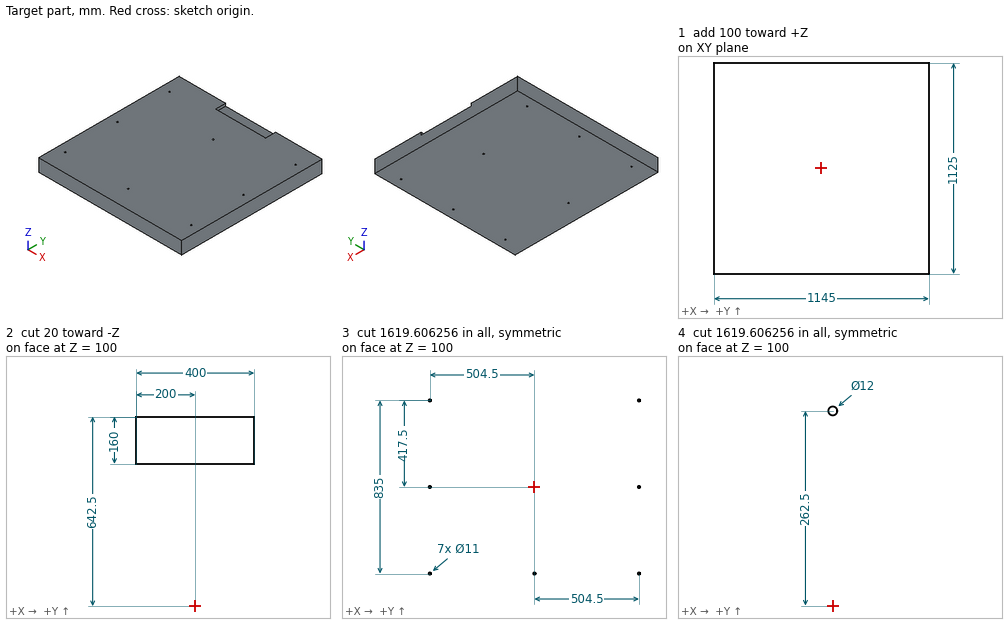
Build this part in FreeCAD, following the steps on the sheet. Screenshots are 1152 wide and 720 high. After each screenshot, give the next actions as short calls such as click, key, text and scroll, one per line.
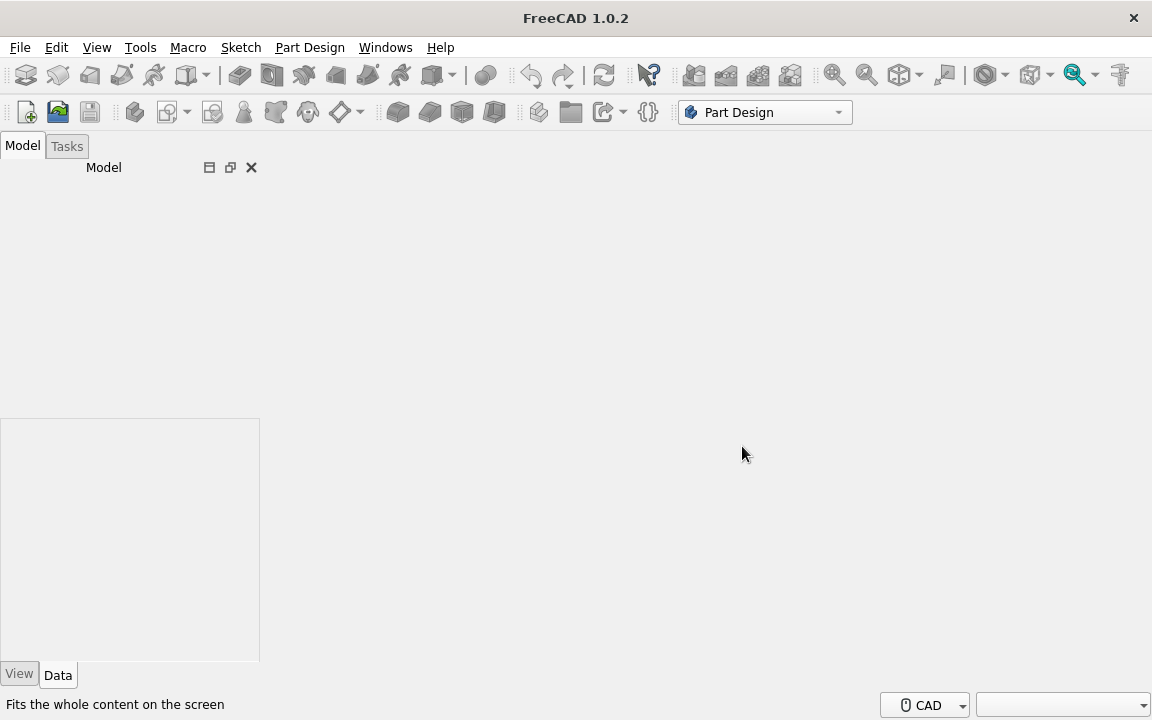
click(26, 112)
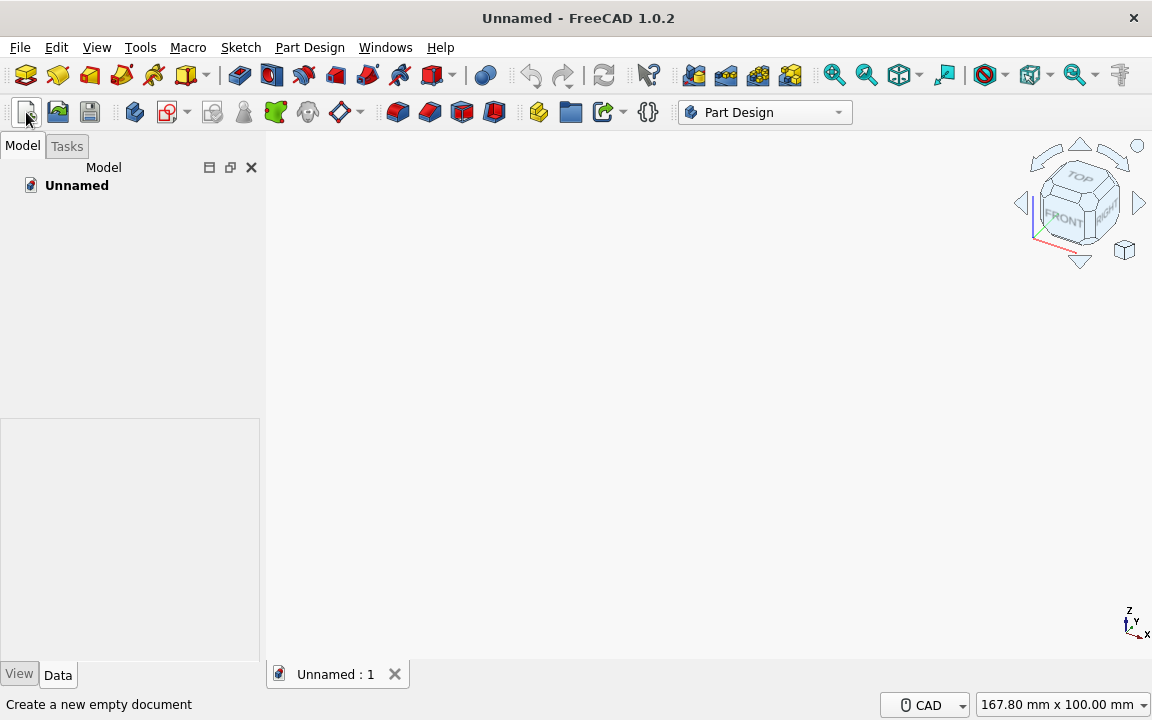
click(168, 112)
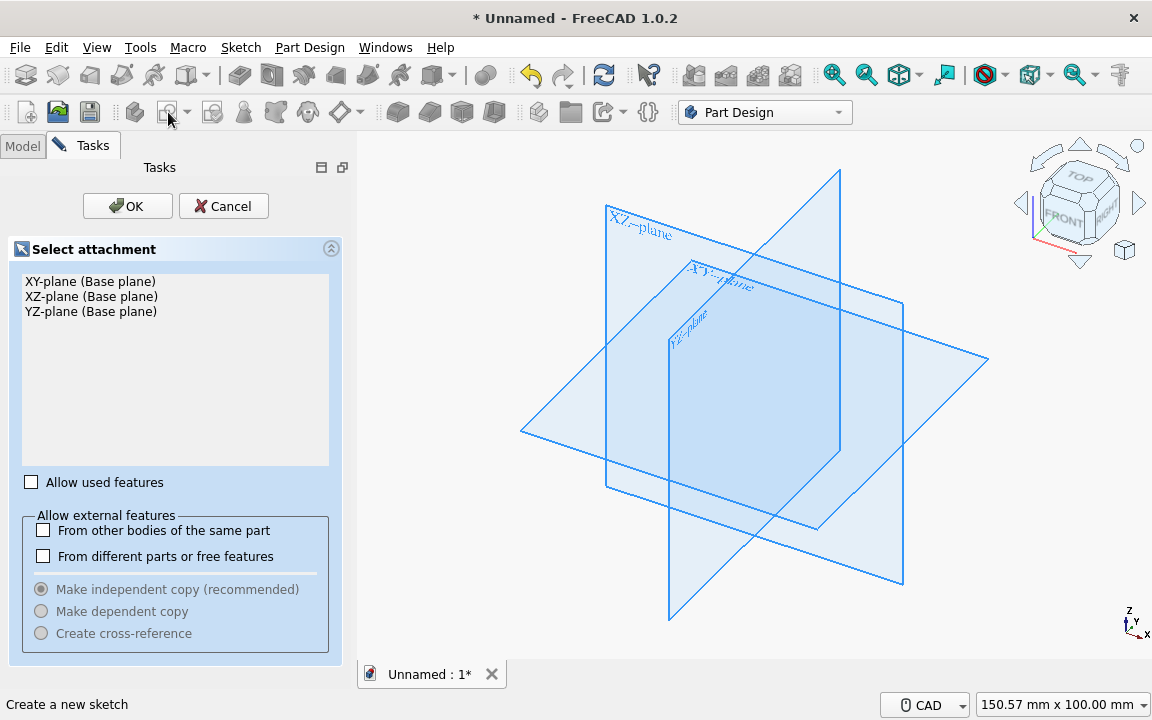
click(82, 282)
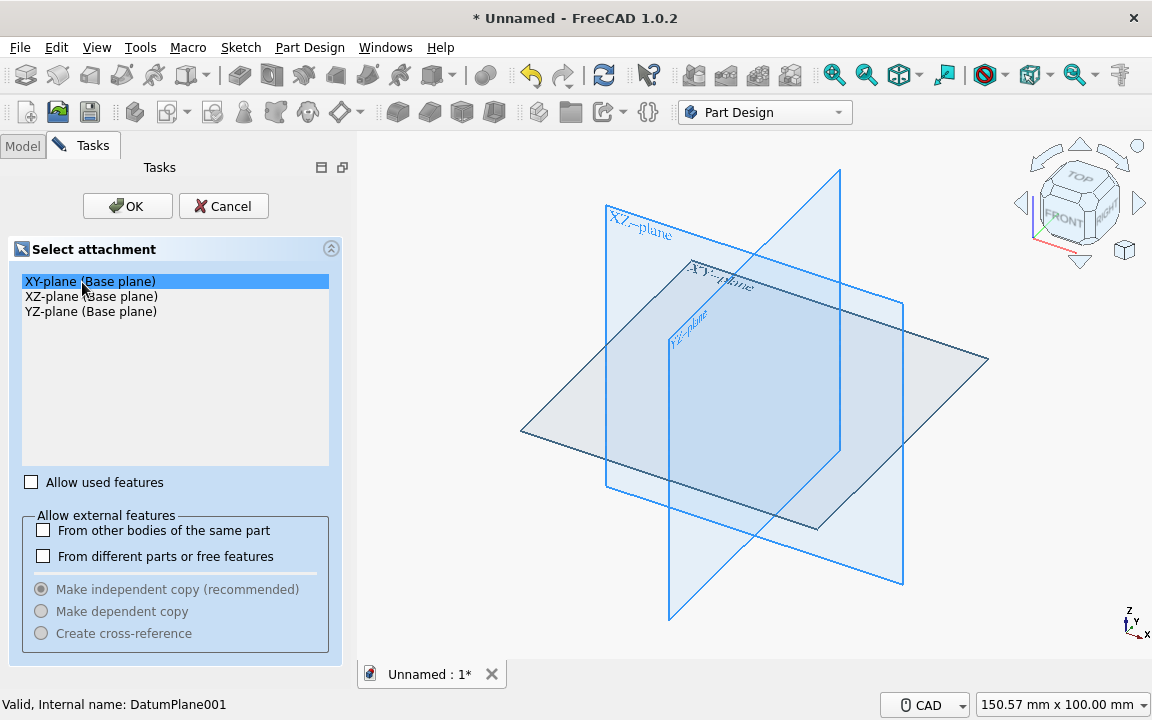
click(128, 206)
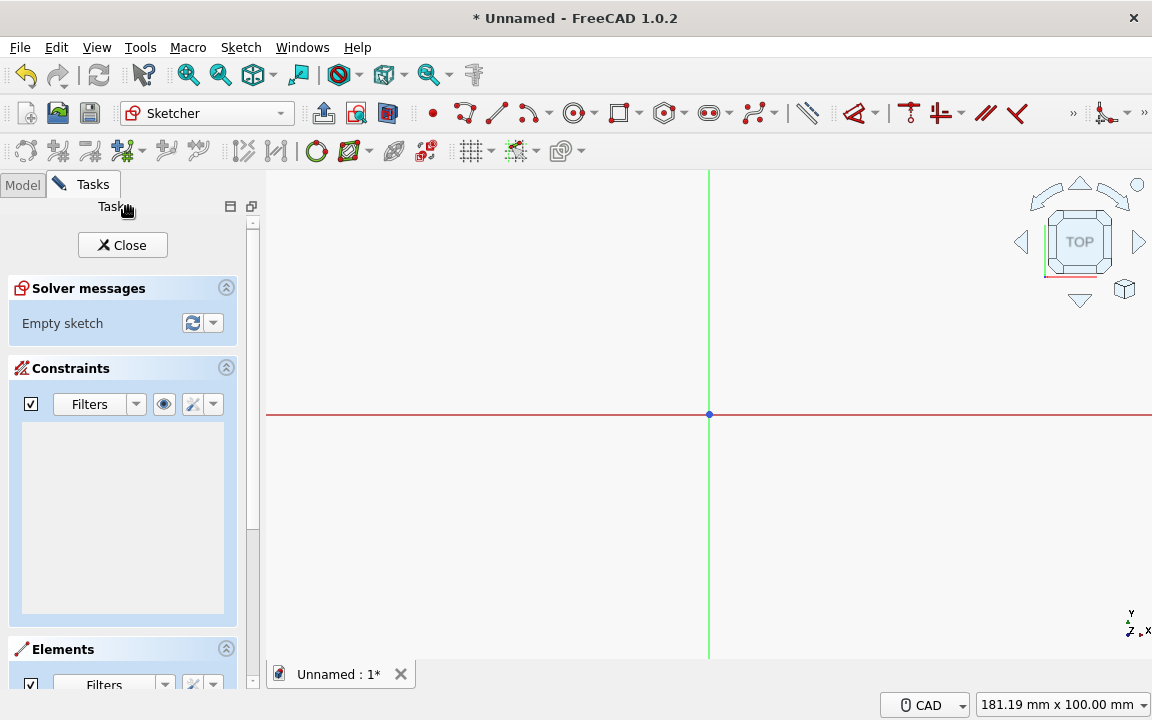
scroll(636, 414, down, 14)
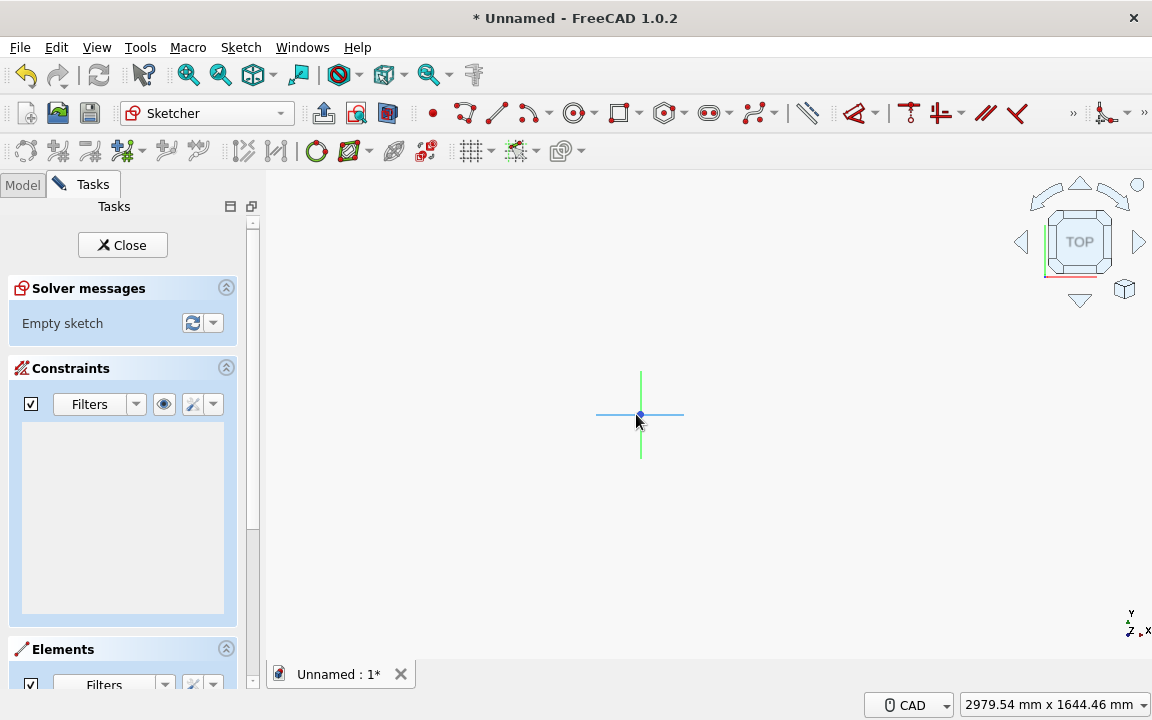
click(642, 114)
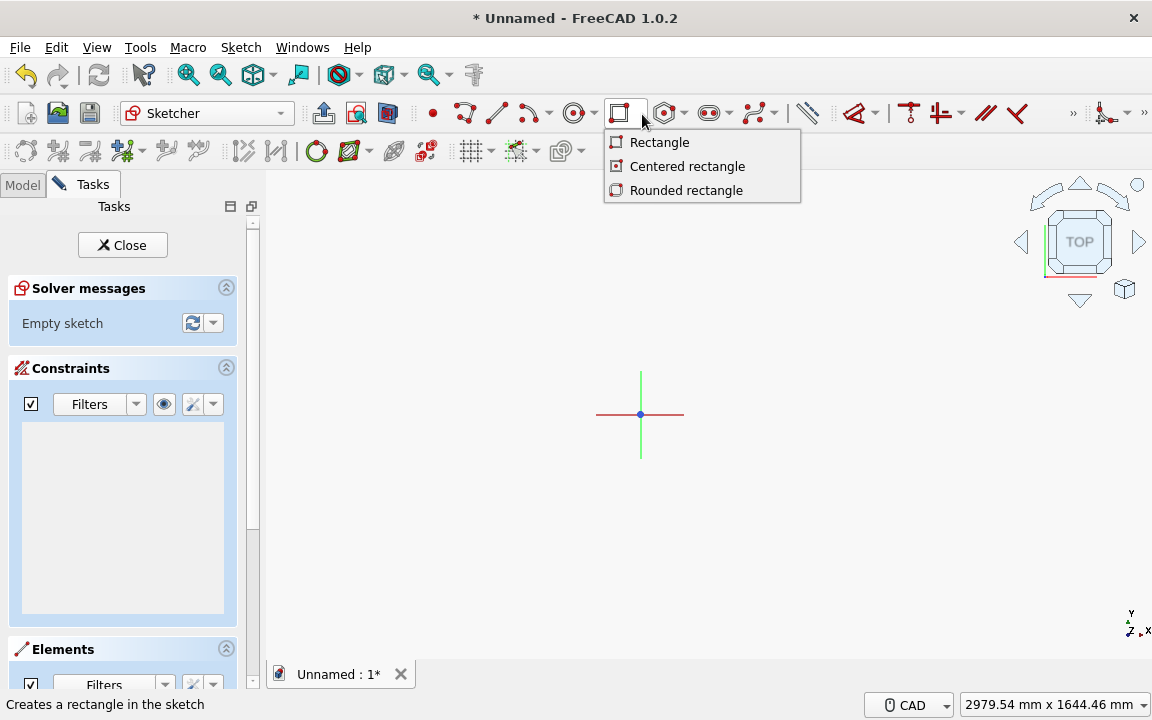
click(702, 166)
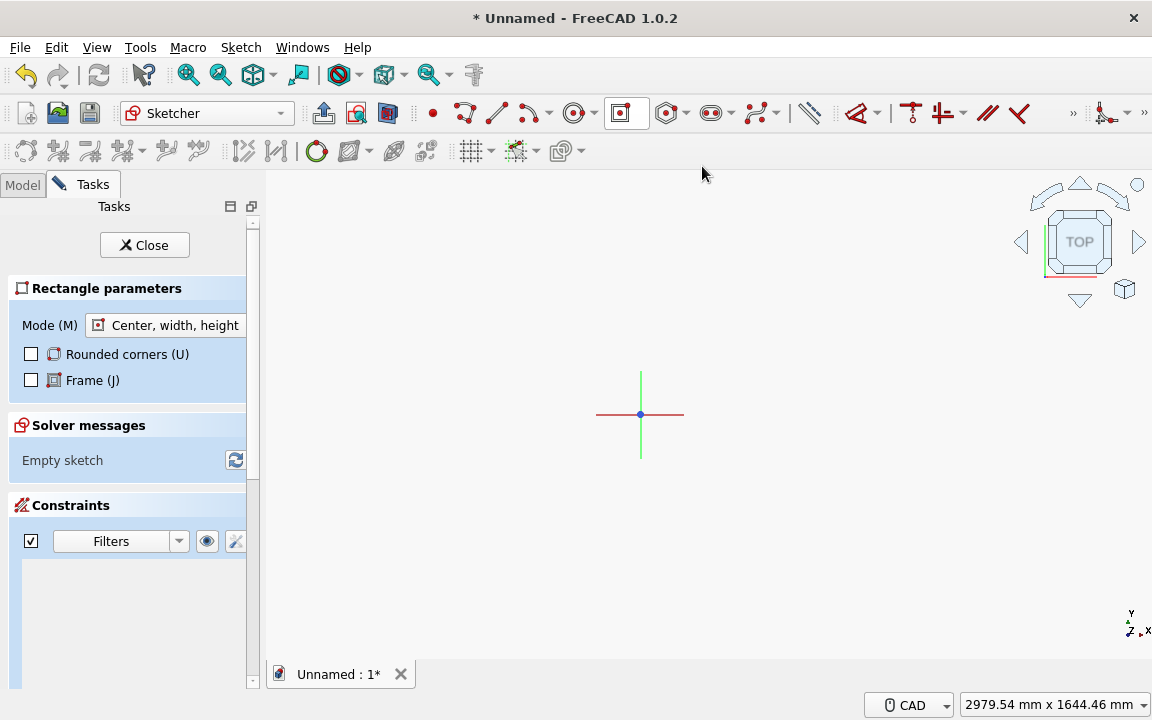
click(641, 414)
click(811, 247)
key(Escape)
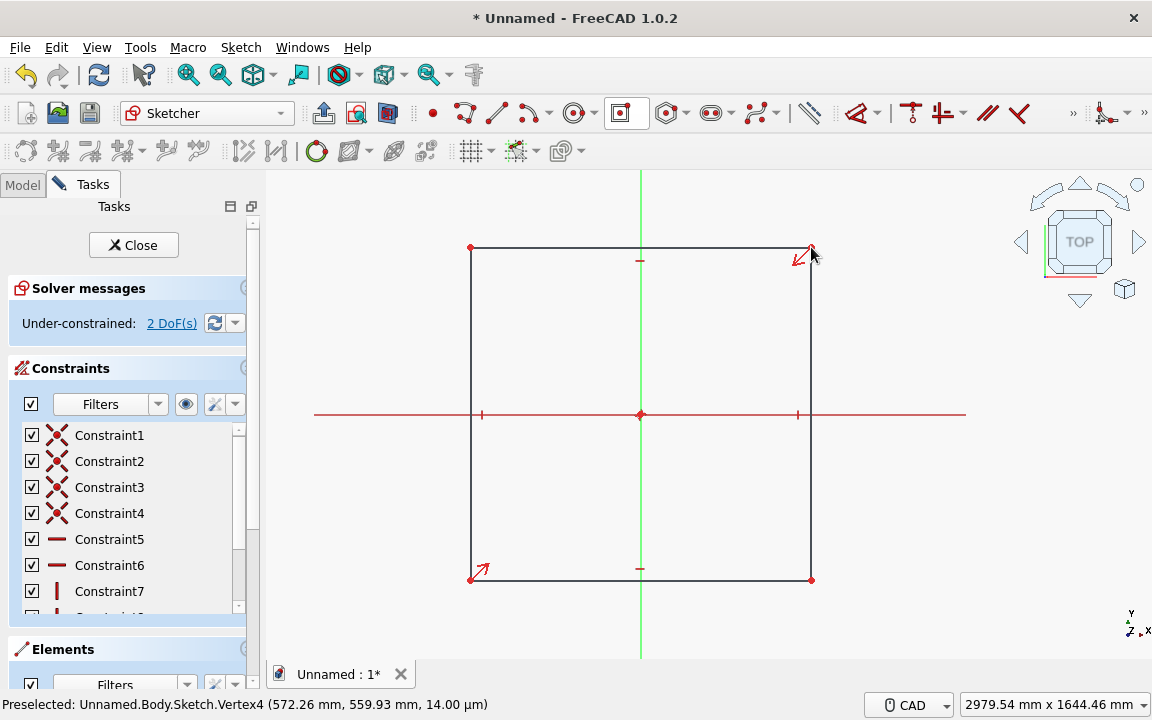
key(d)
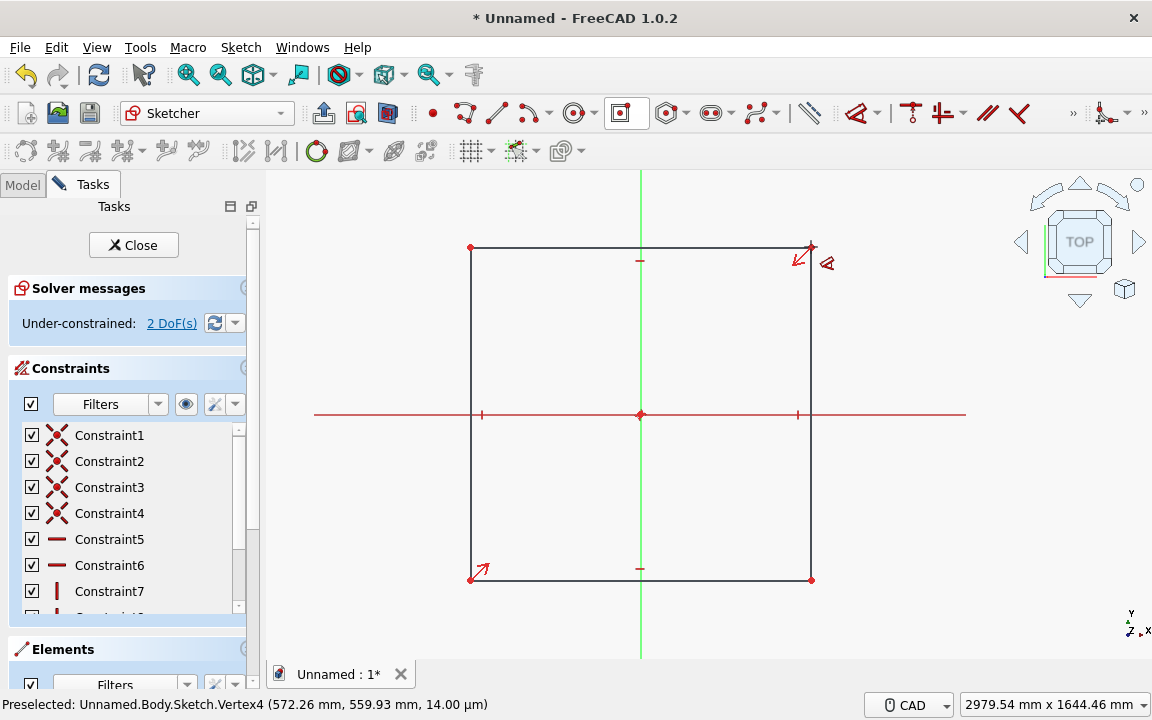
click(573, 581)
click(563, 615)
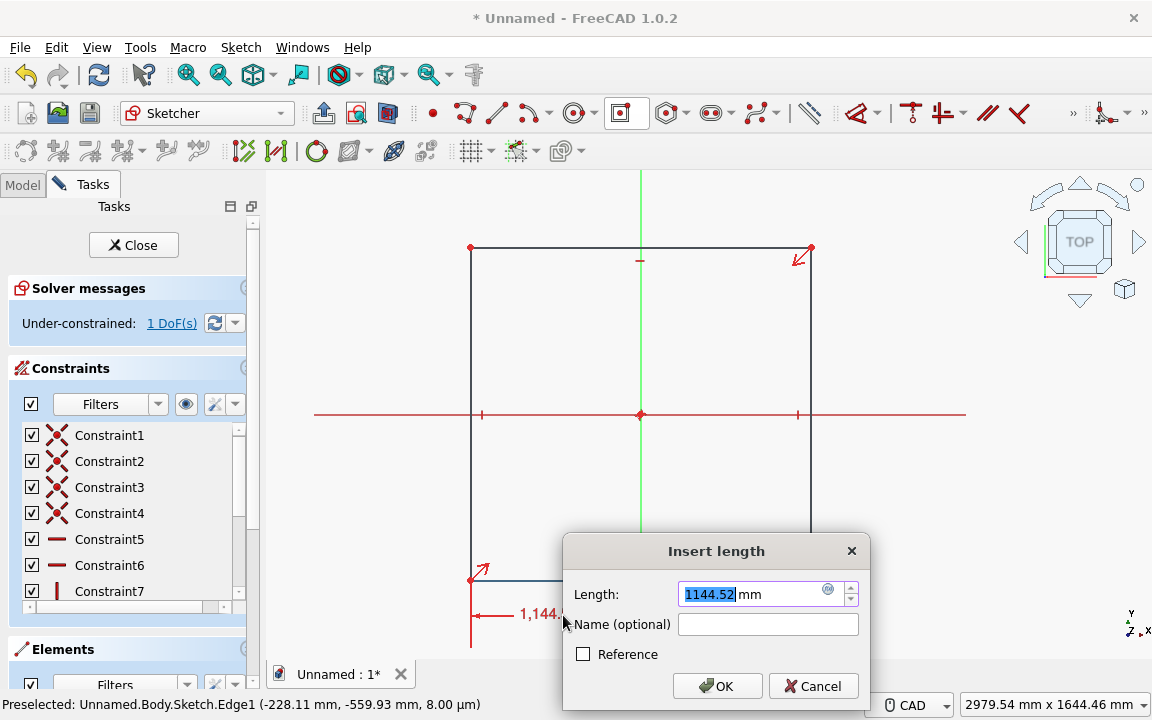
text(1145)
key(Return)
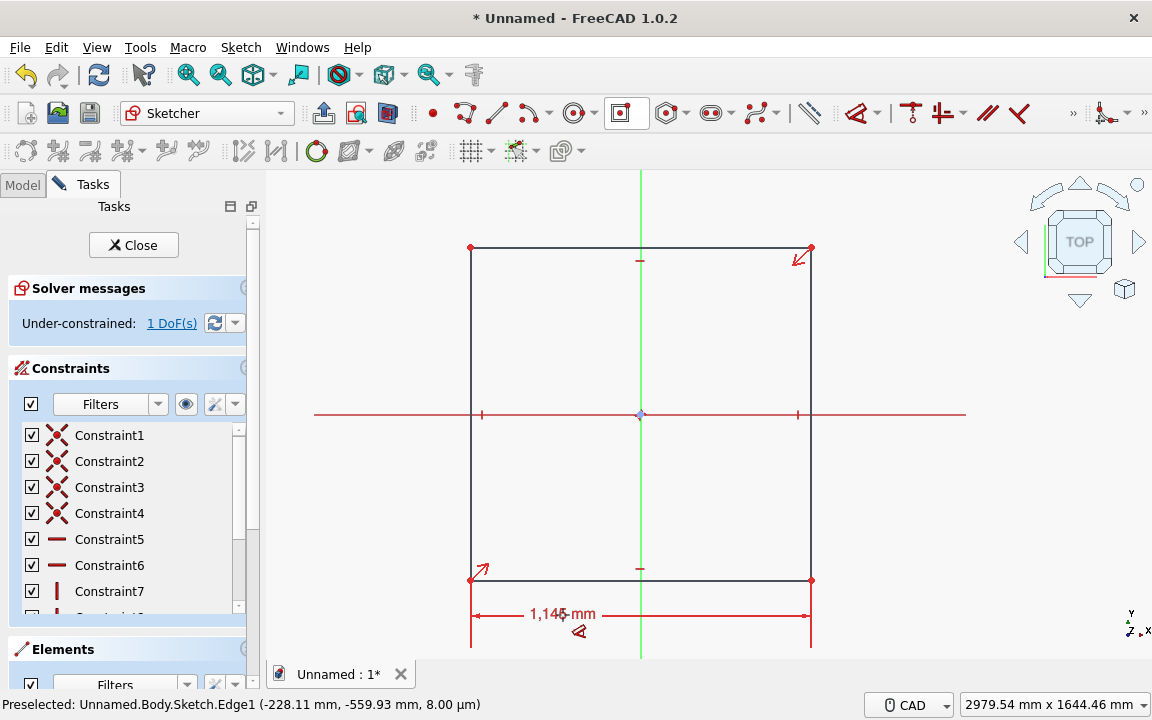
click(811, 481)
click(845, 338)